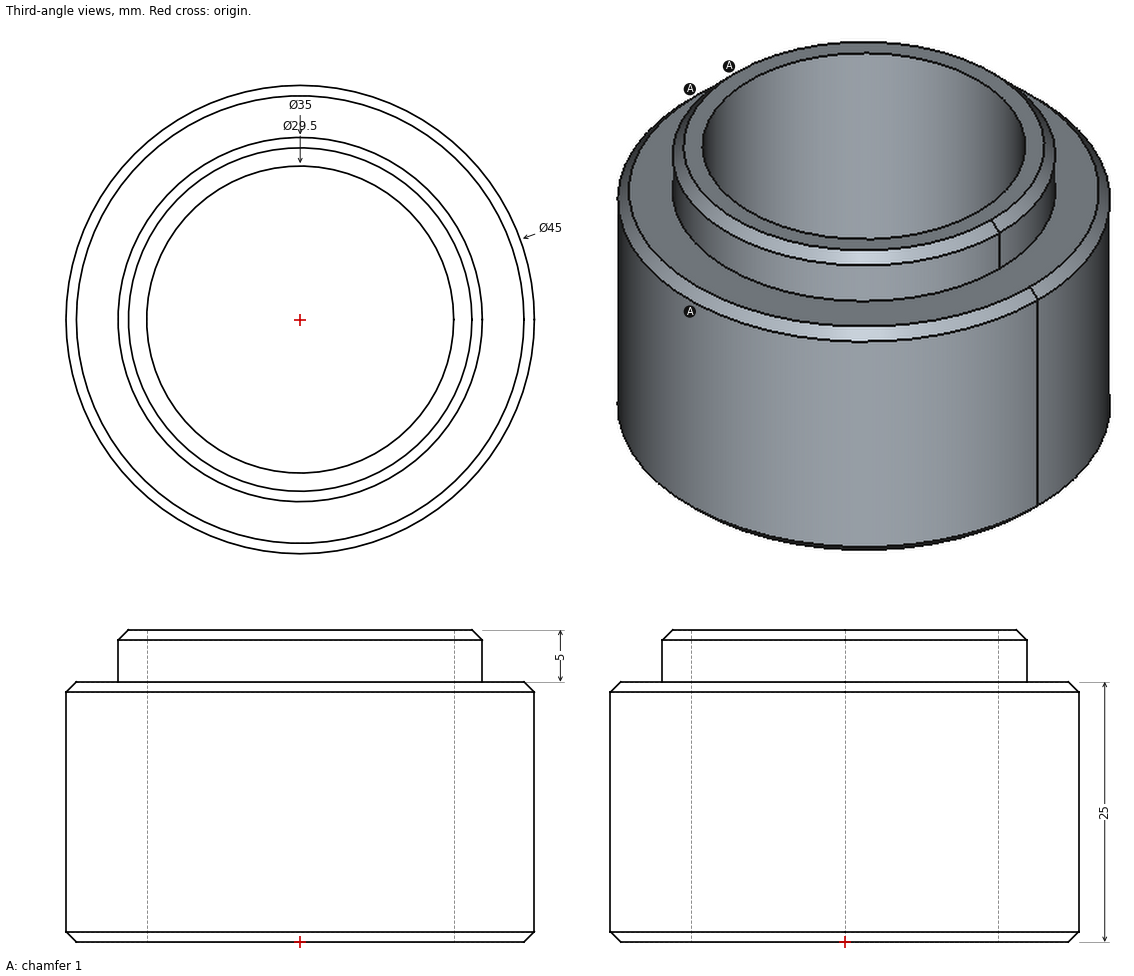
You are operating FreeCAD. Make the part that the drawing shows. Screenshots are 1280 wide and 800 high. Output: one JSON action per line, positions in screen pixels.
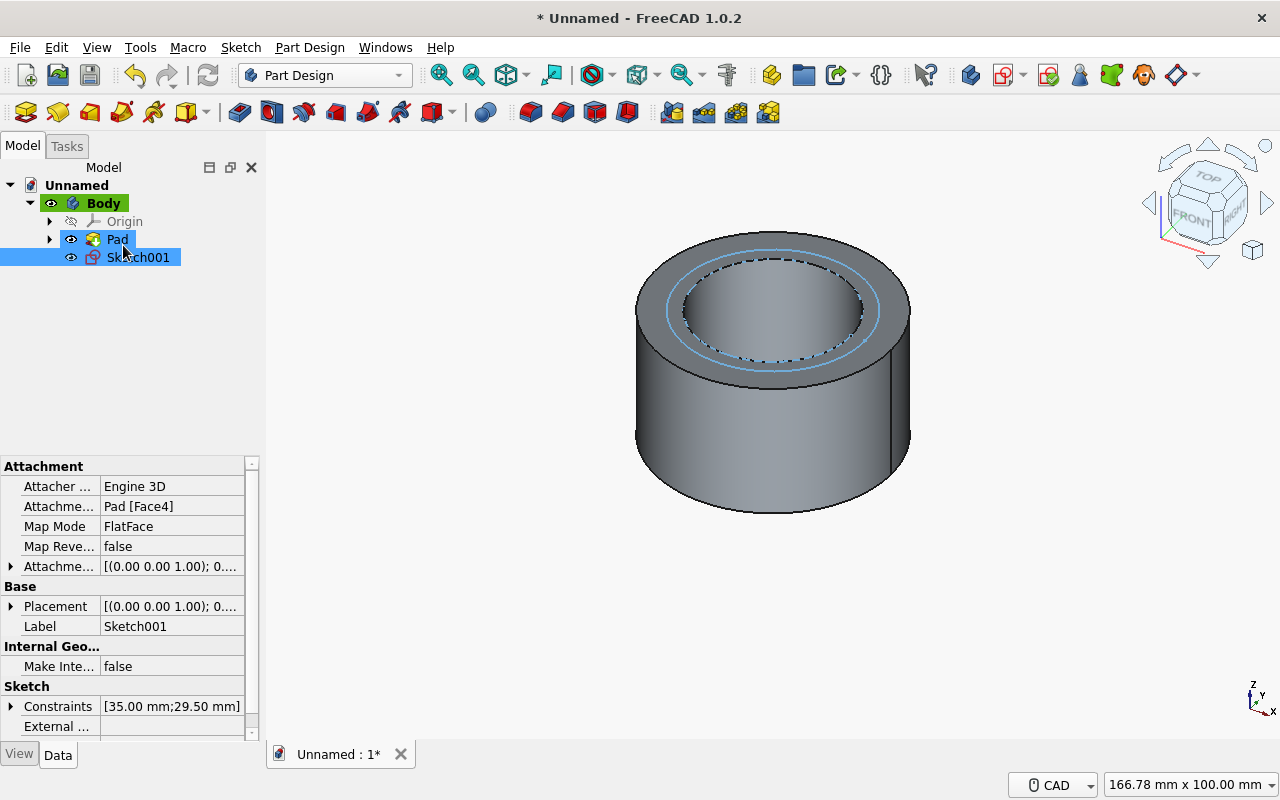
{"action": "left_click", "coordinate": [26, 112]}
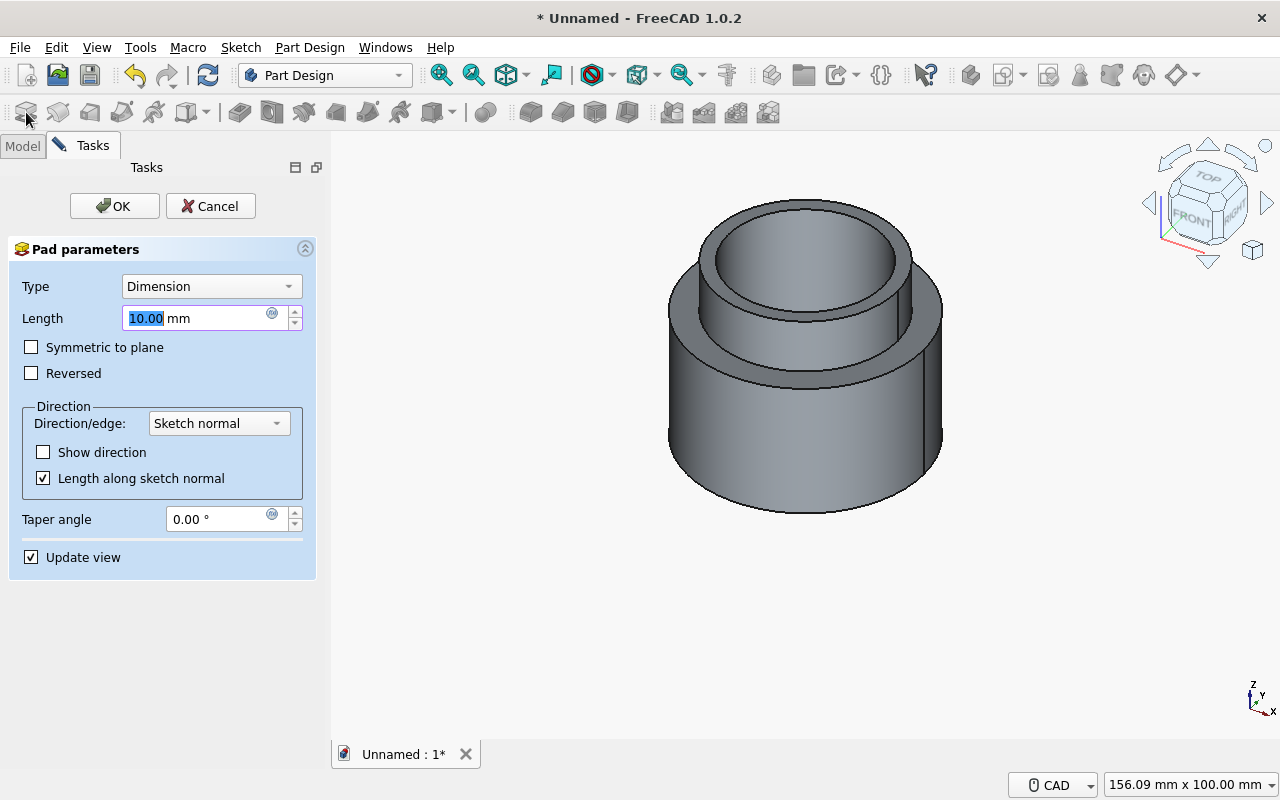
{"action": "type", "text": "5"}
{"action": "key", "text": "Tab"}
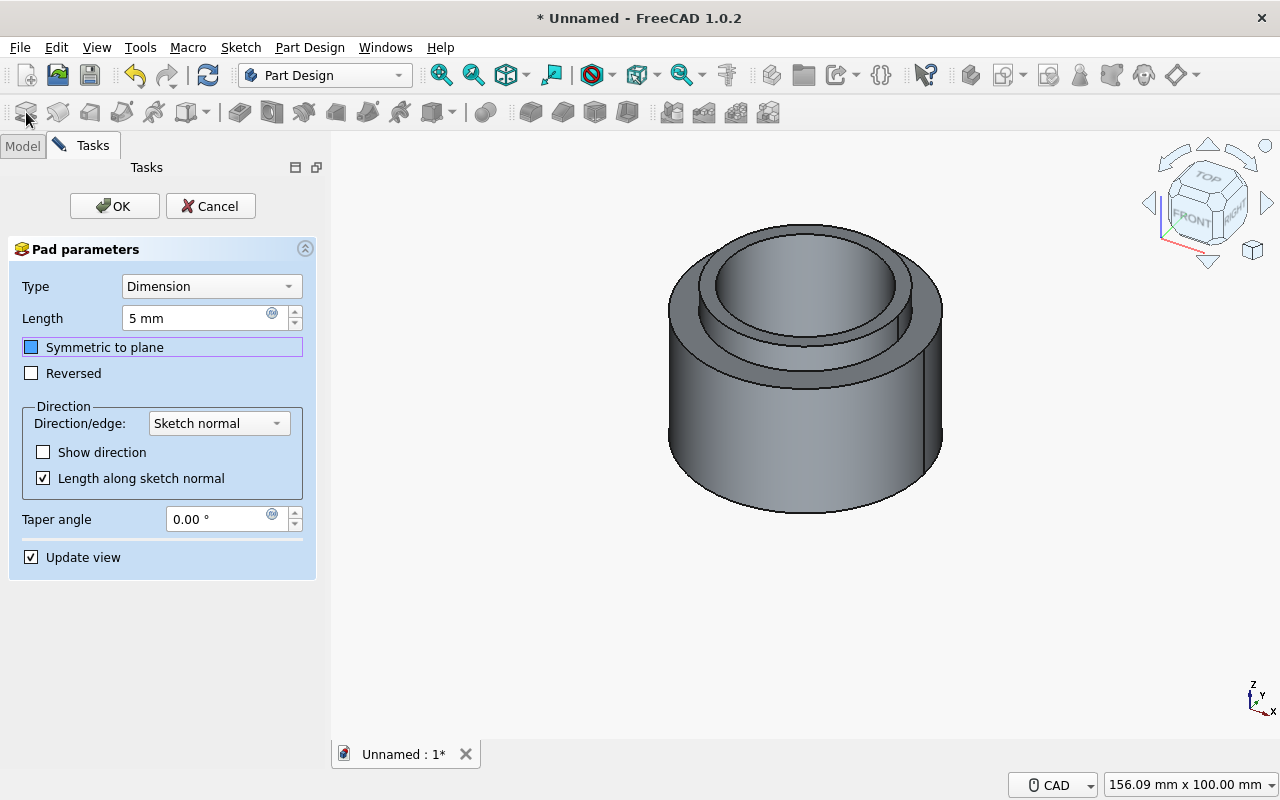
{"action": "left_click", "coordinate": [115, 206]}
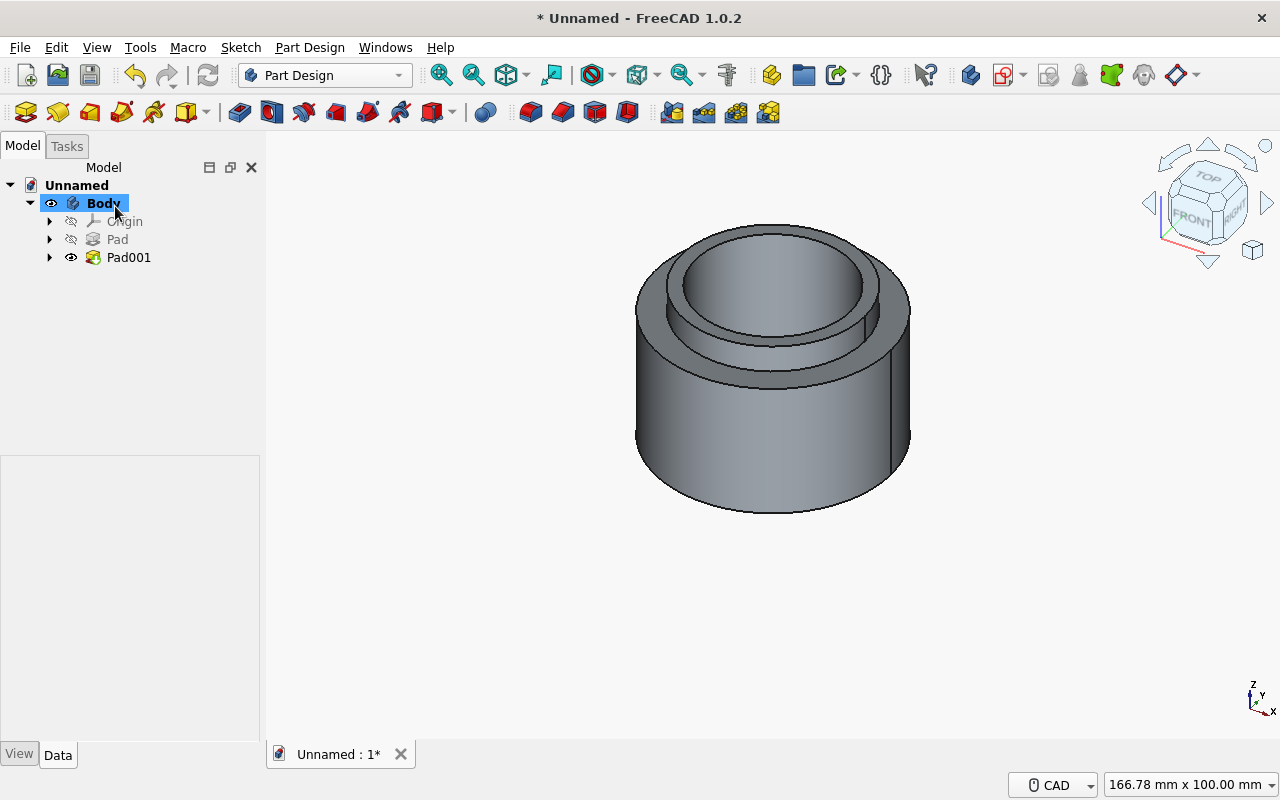
{"action": "left_click", "coordinate": [667, 291]}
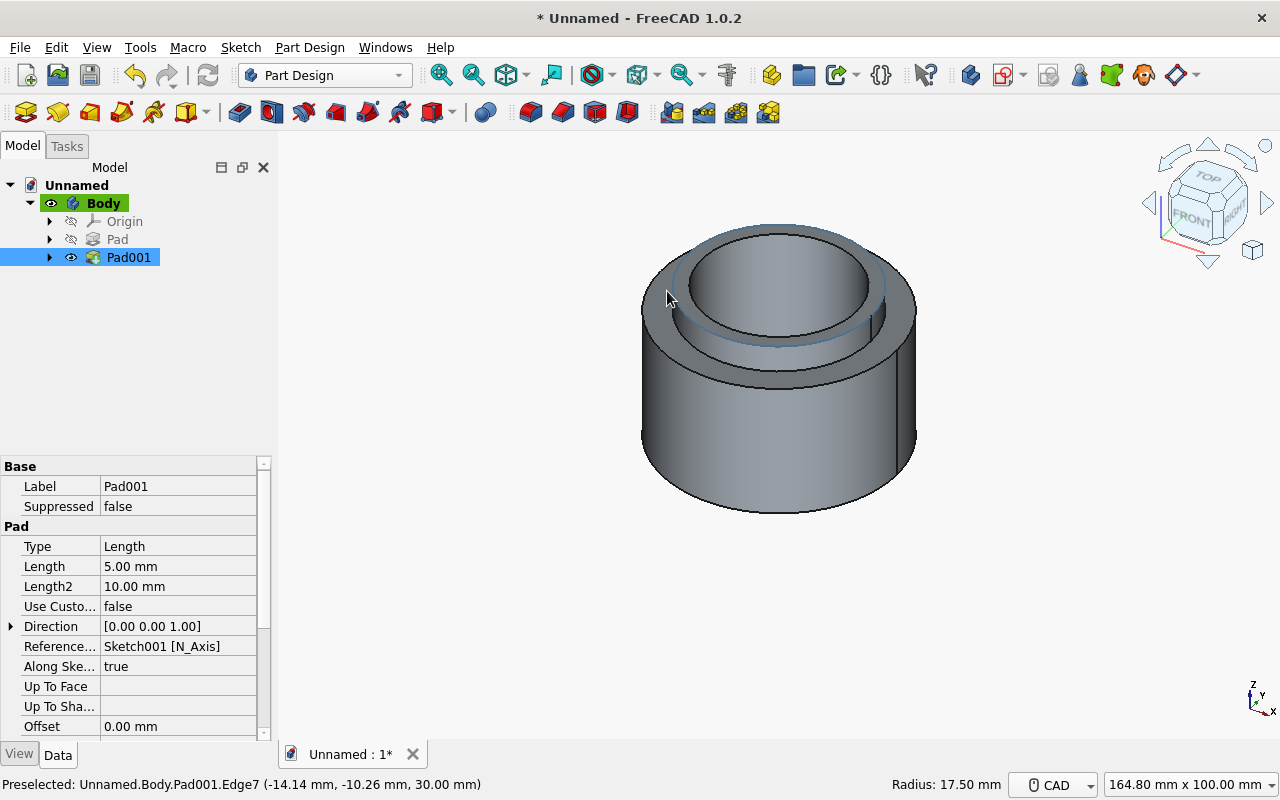
{"action": "left_click", "coordinate": [677, 487], "text": "ctrl"}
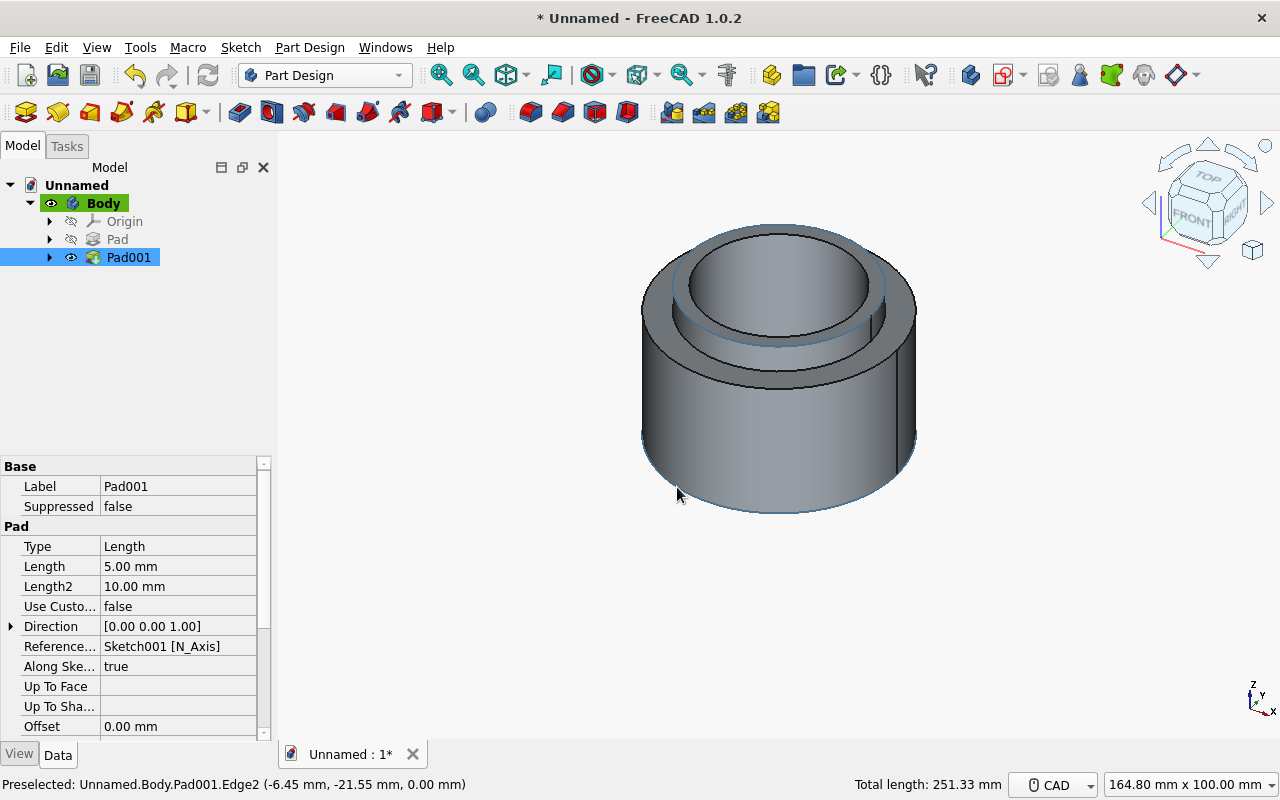
{"action": "left_click", "coordinate": [643, 318], "text": "ctrl"}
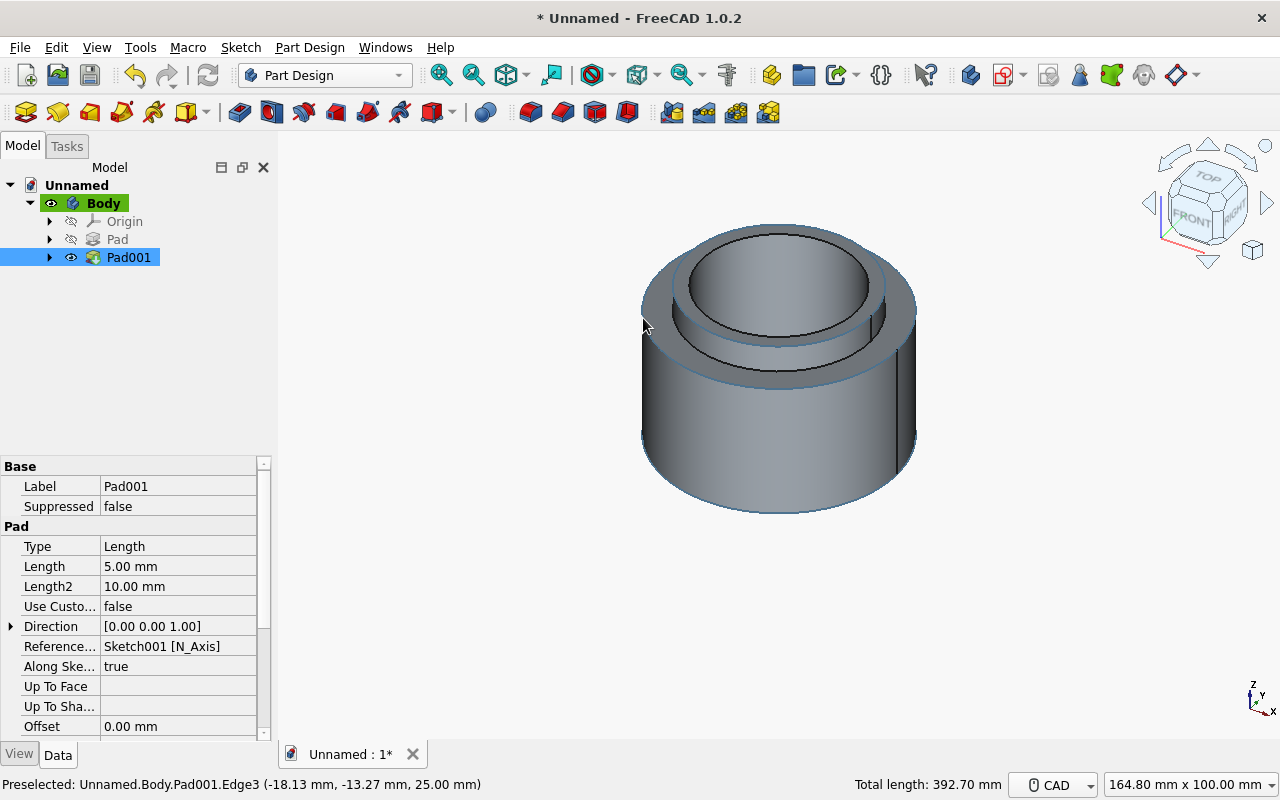
{"action": "left_click", "coordinate": [564, 112]}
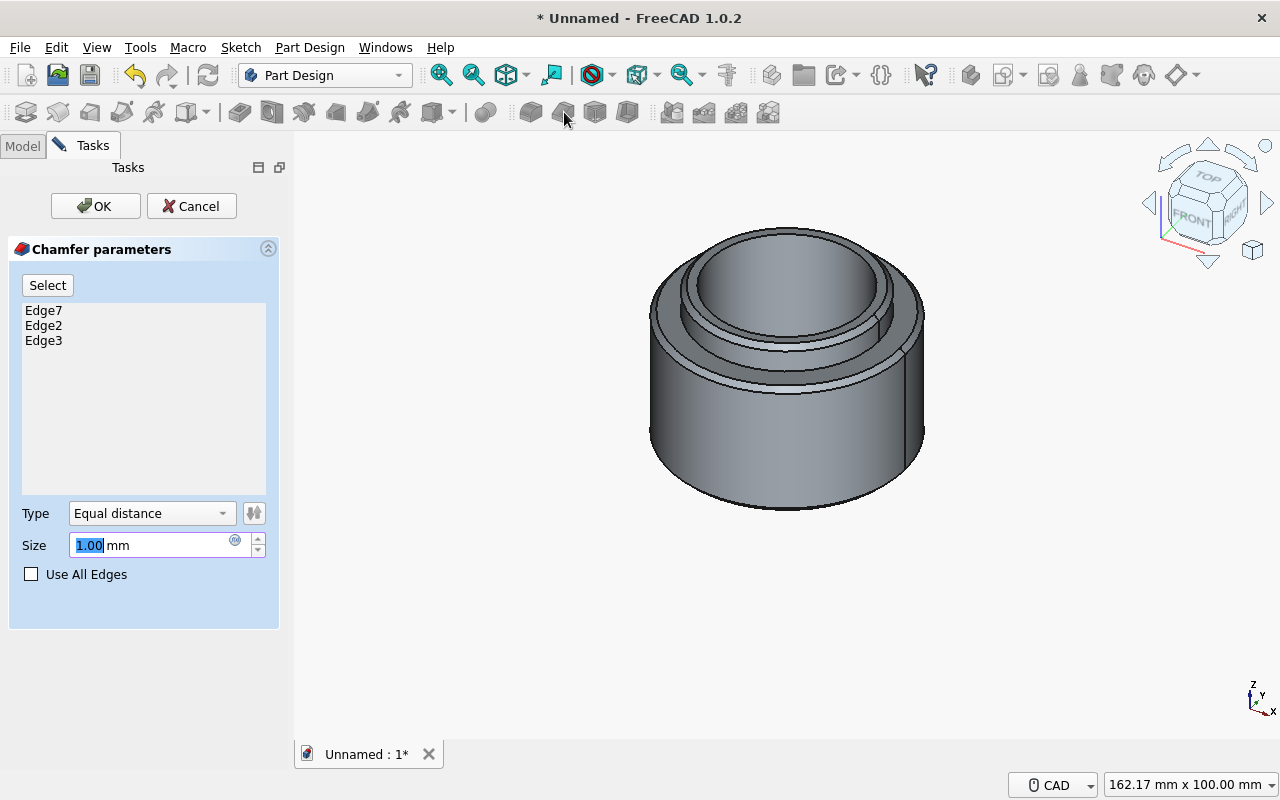
{"action": "type", "text": "1"}
{"action": "key", "text": "Tab"}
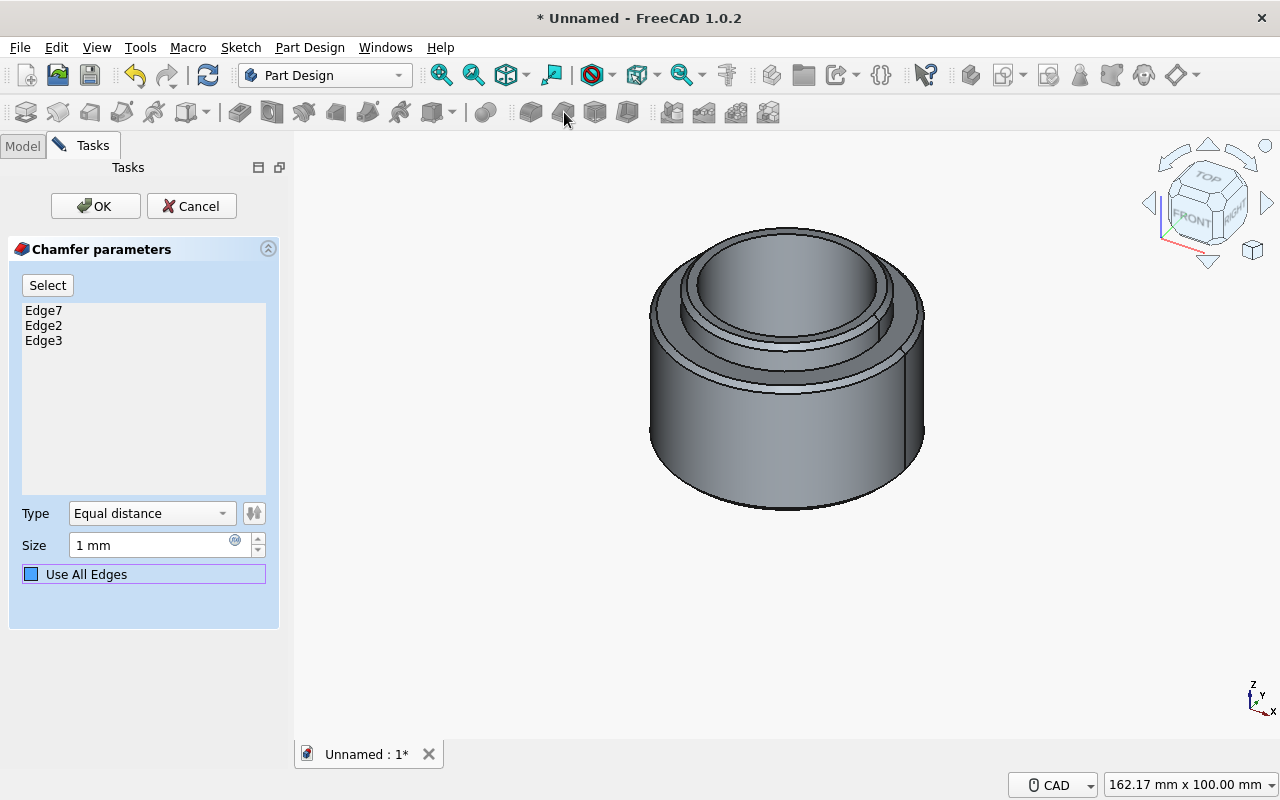
{"action": "left_click", "coordinate": [96, 206]}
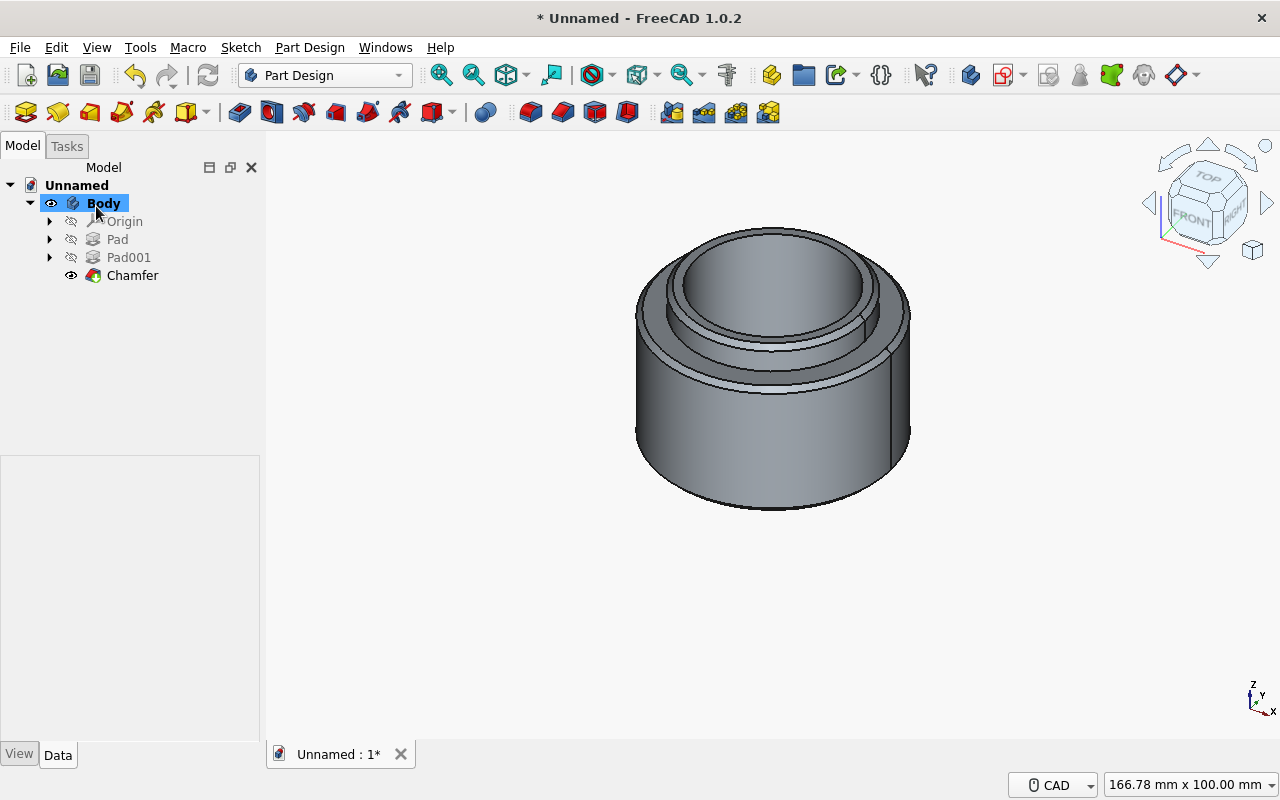
{"action": "key", "text": "0"}